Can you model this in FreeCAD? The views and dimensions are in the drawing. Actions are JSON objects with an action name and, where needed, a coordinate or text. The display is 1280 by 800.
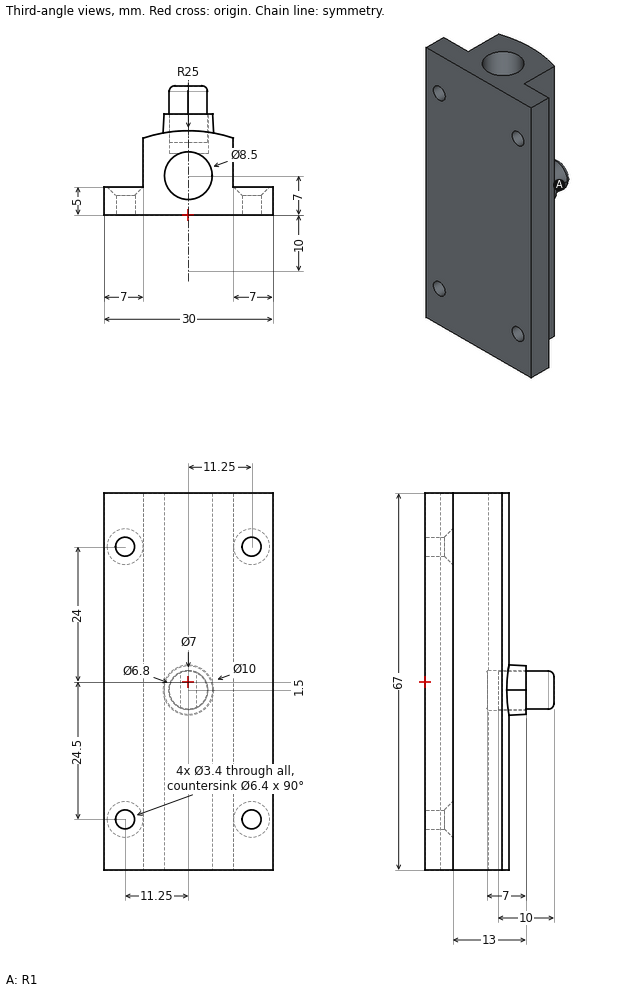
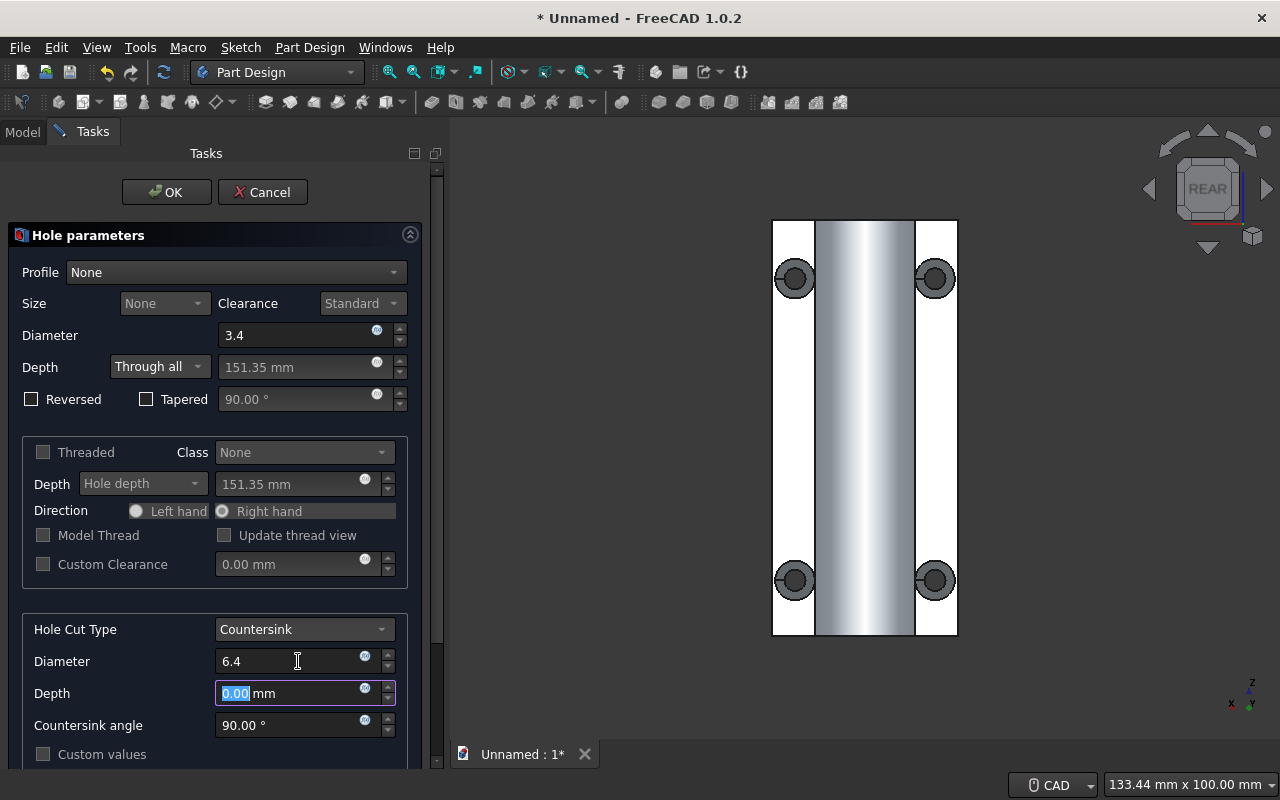
{"action": "left_click", "coordinate": [167, 192]}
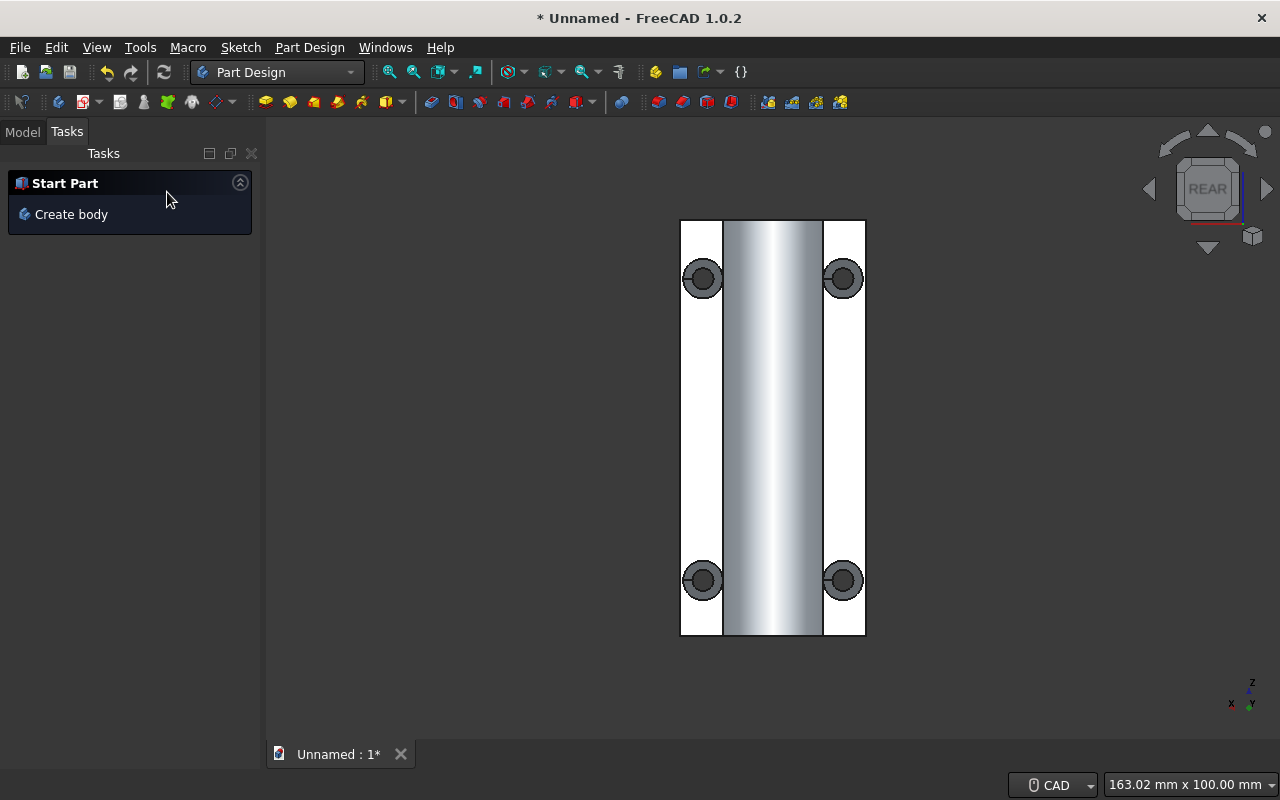
{"action": "left_click", "coordinate": [701, 367]}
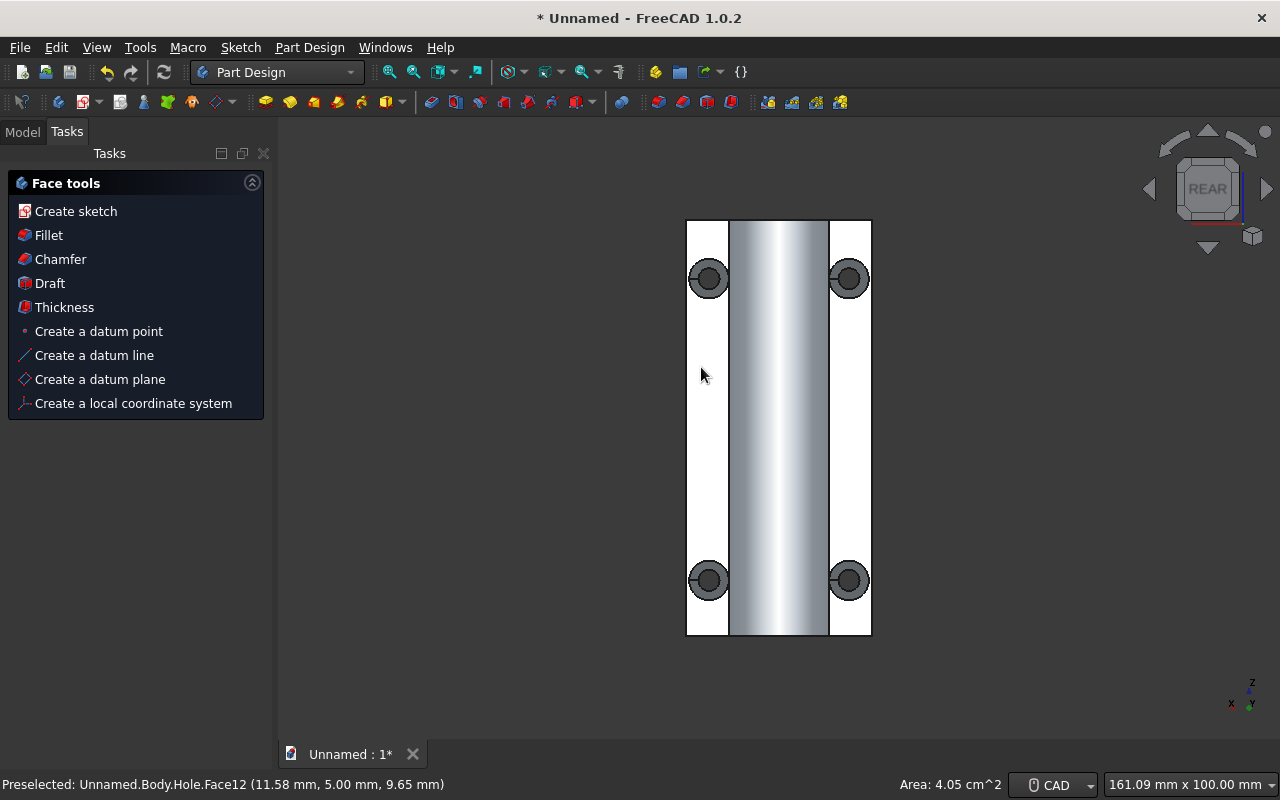
{"action": "left_click", "coordinate": [84, 102]}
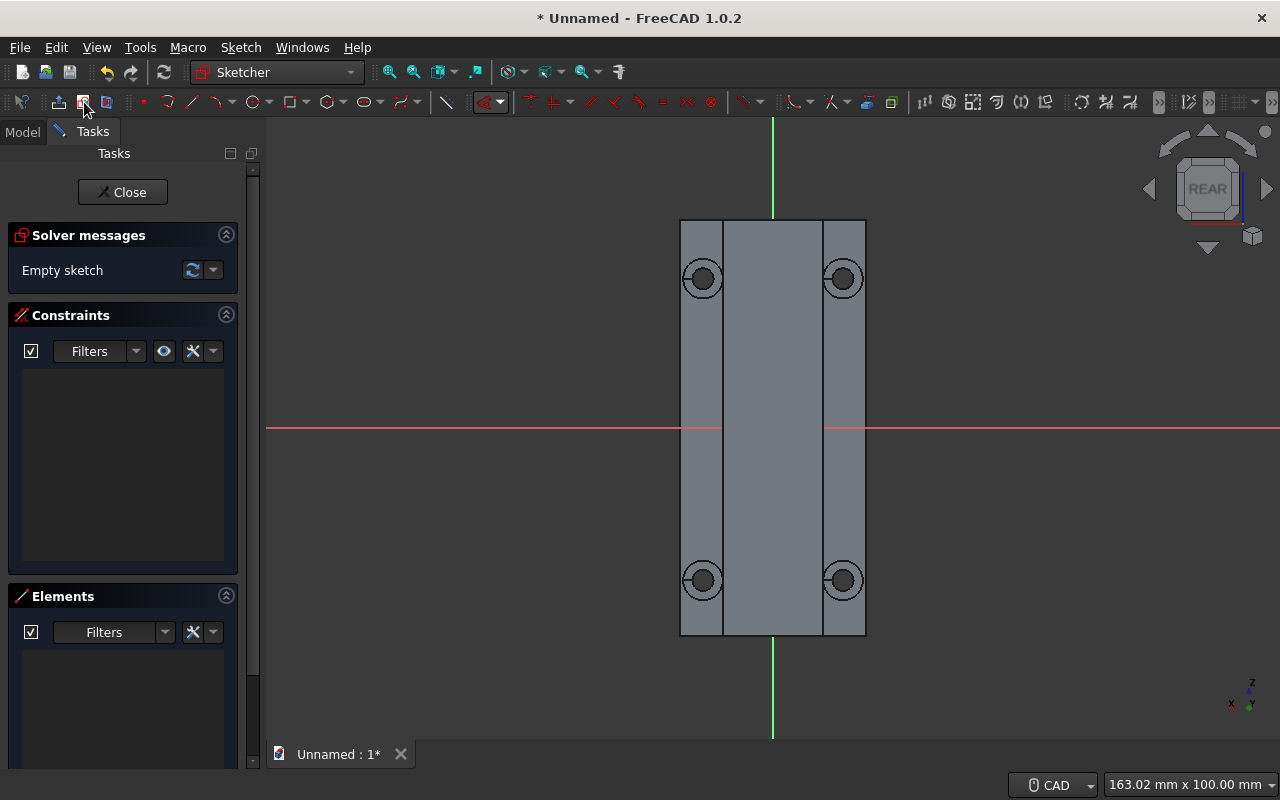
{"action": "scroll", "coordinate": [787, 439], "scroll_direction": "up", "scroll_amount": 9}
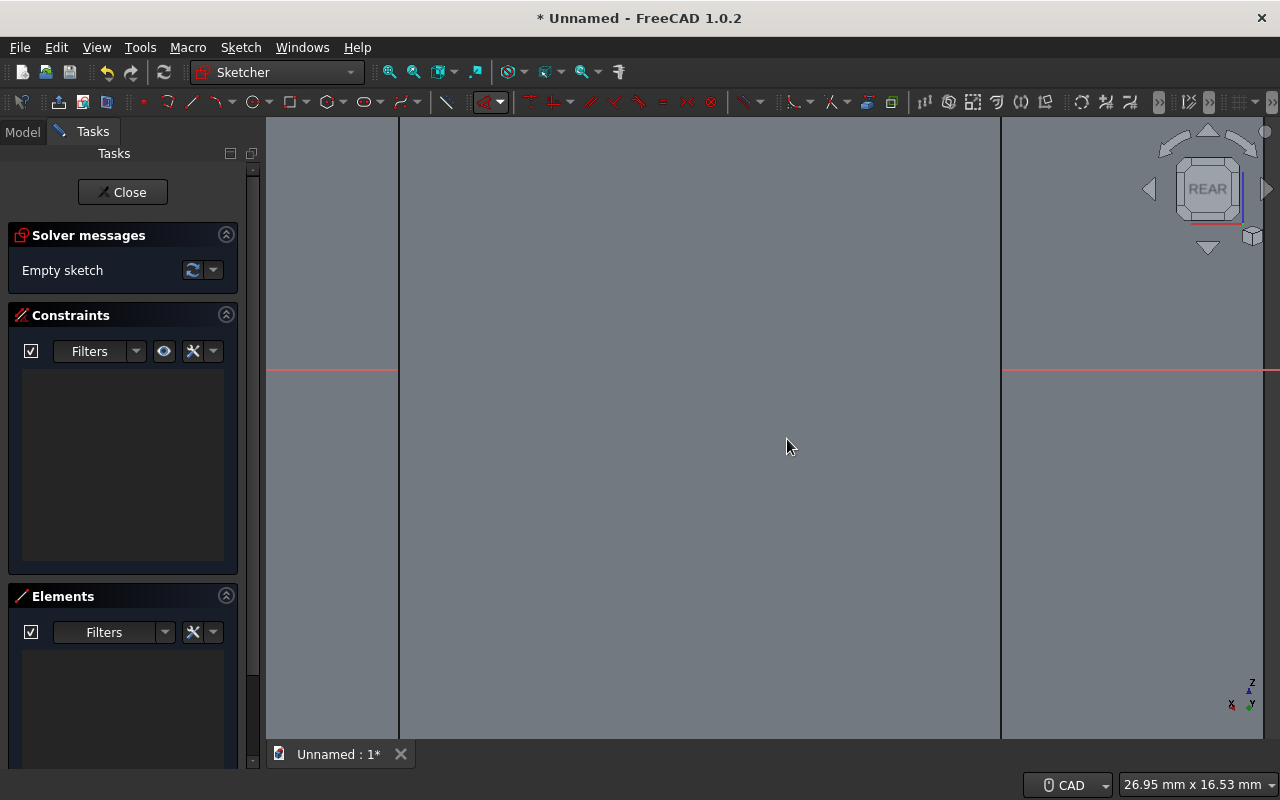
{"action": "left_click", "coordinate": [254, 102]}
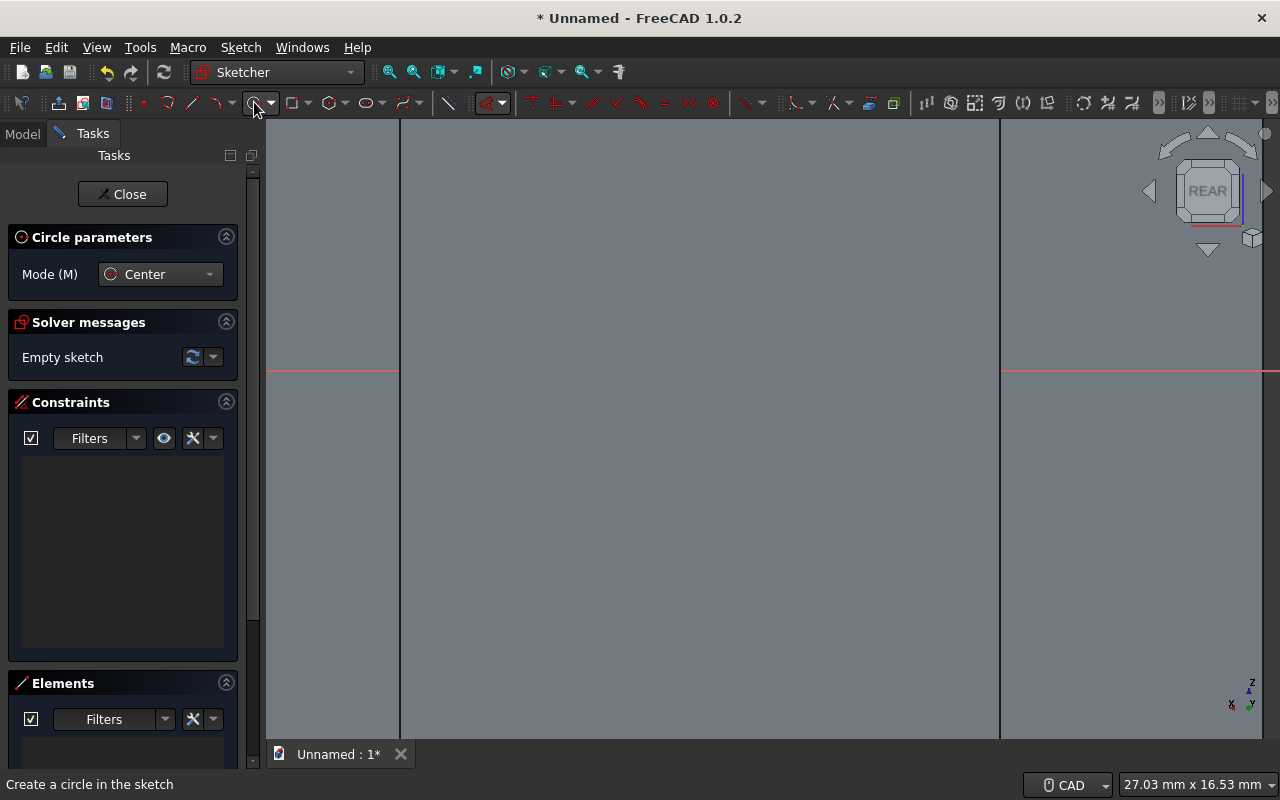
{"action": "left_click", "coordinate": [700, 427]}
{"action": "left_click", "coordinate": [833, 295]}
{"action": "key", "text": "Escape"}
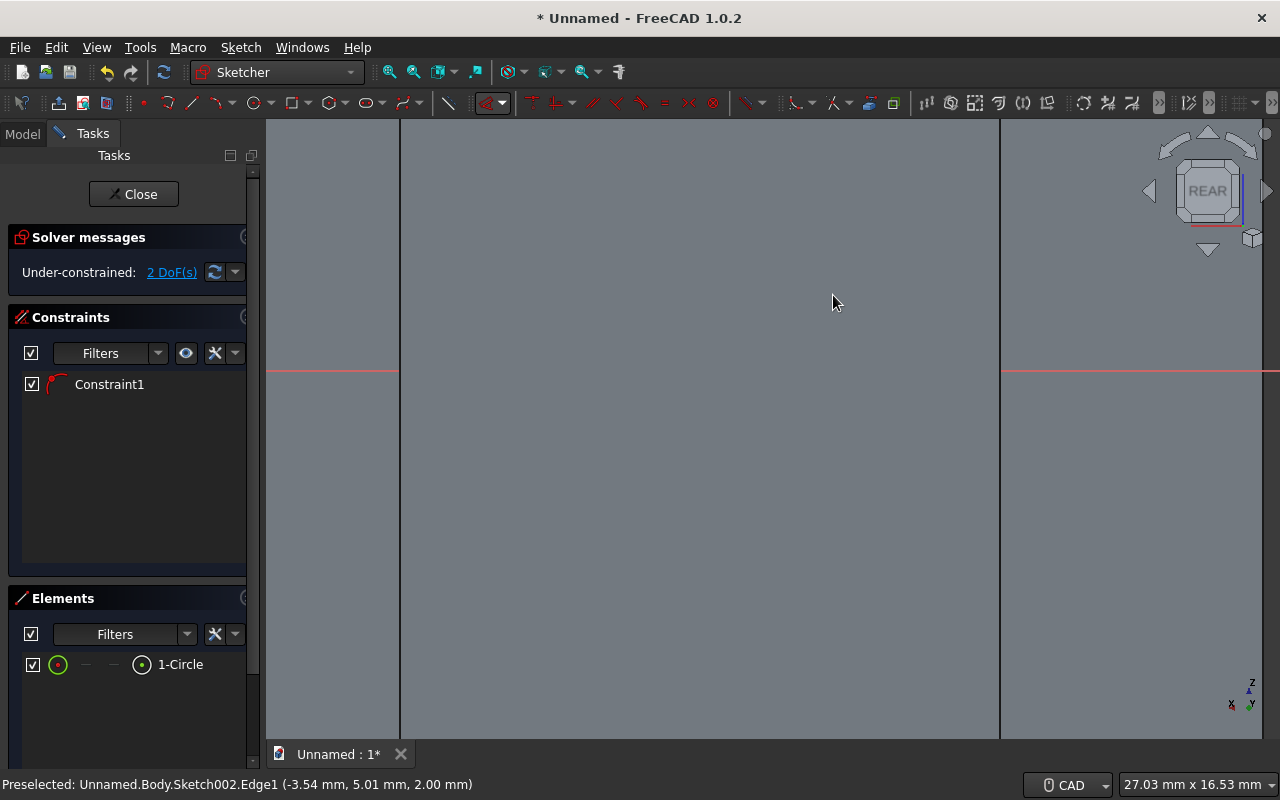
{"action": "left_click", "coordinate": [832, 295]}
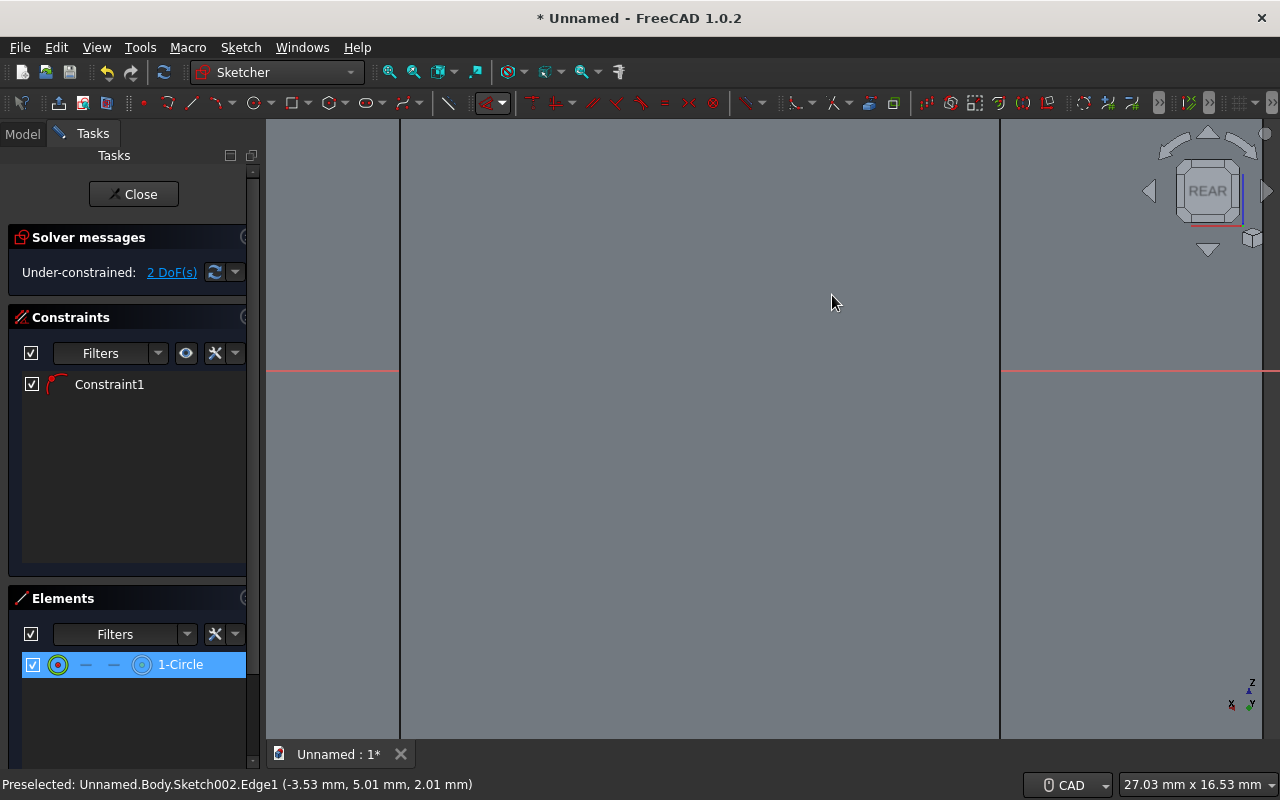
{"action": "key", "text": "k o"}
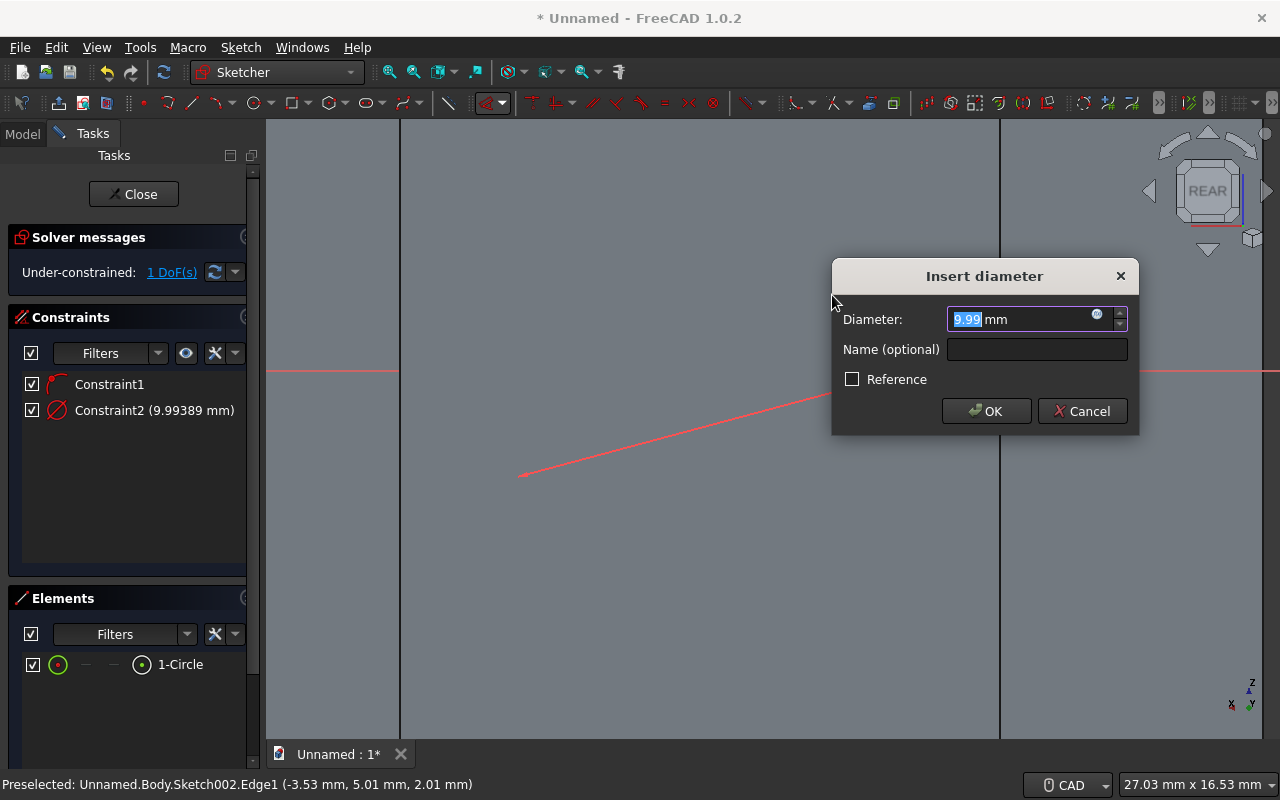
{"action": "type", "text": "10"}
{"action": "key", "text": "Return"}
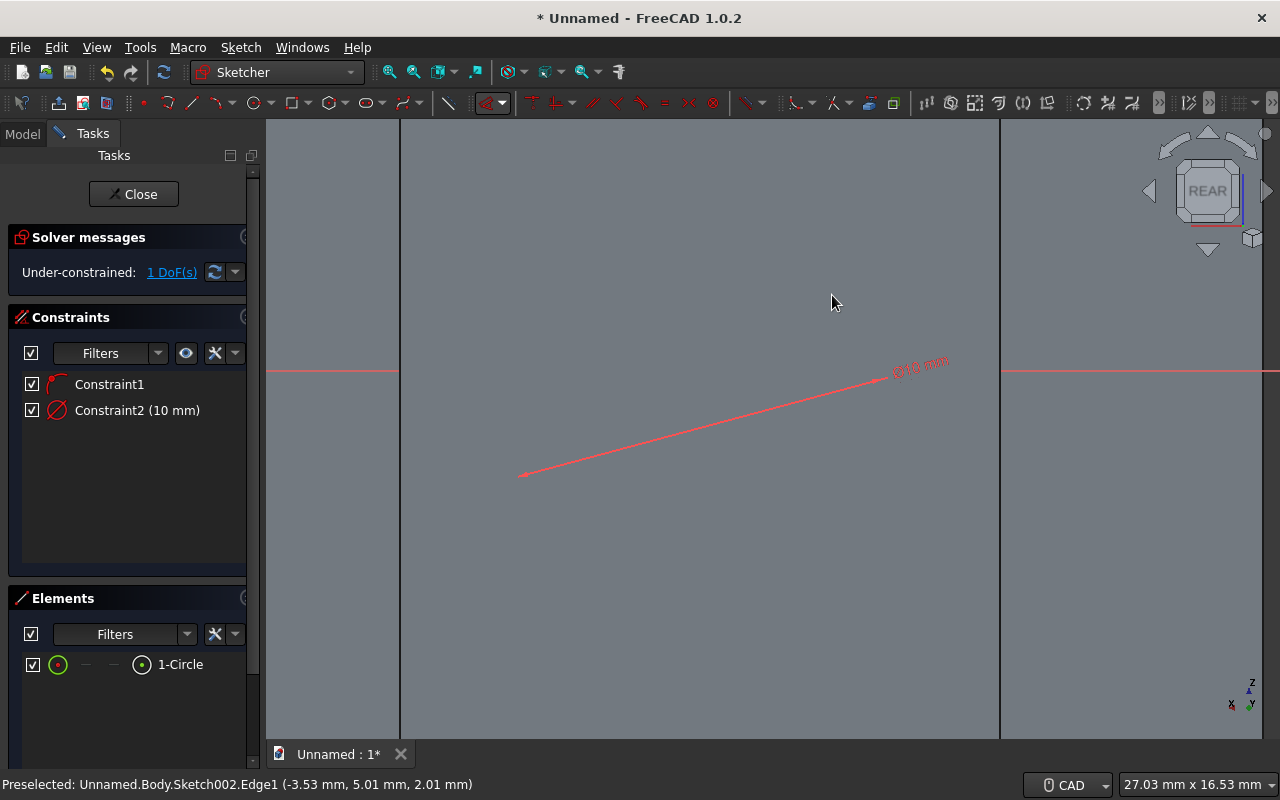
{"action": "left_click", "coordinate": [700, 428]}